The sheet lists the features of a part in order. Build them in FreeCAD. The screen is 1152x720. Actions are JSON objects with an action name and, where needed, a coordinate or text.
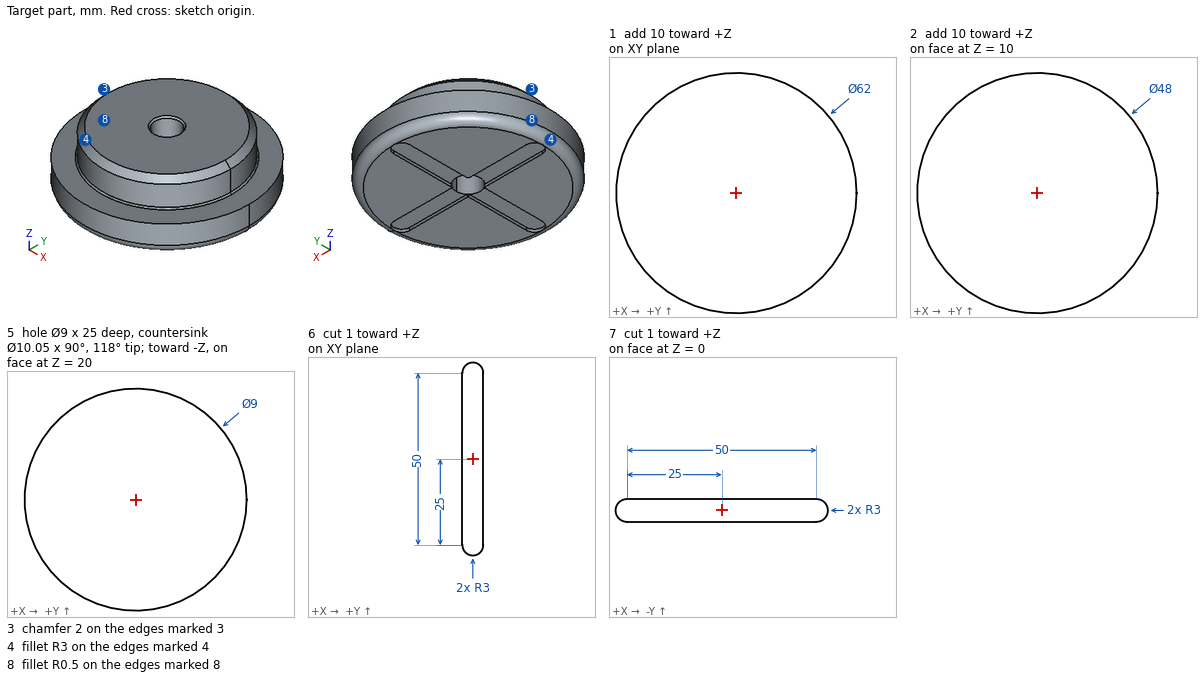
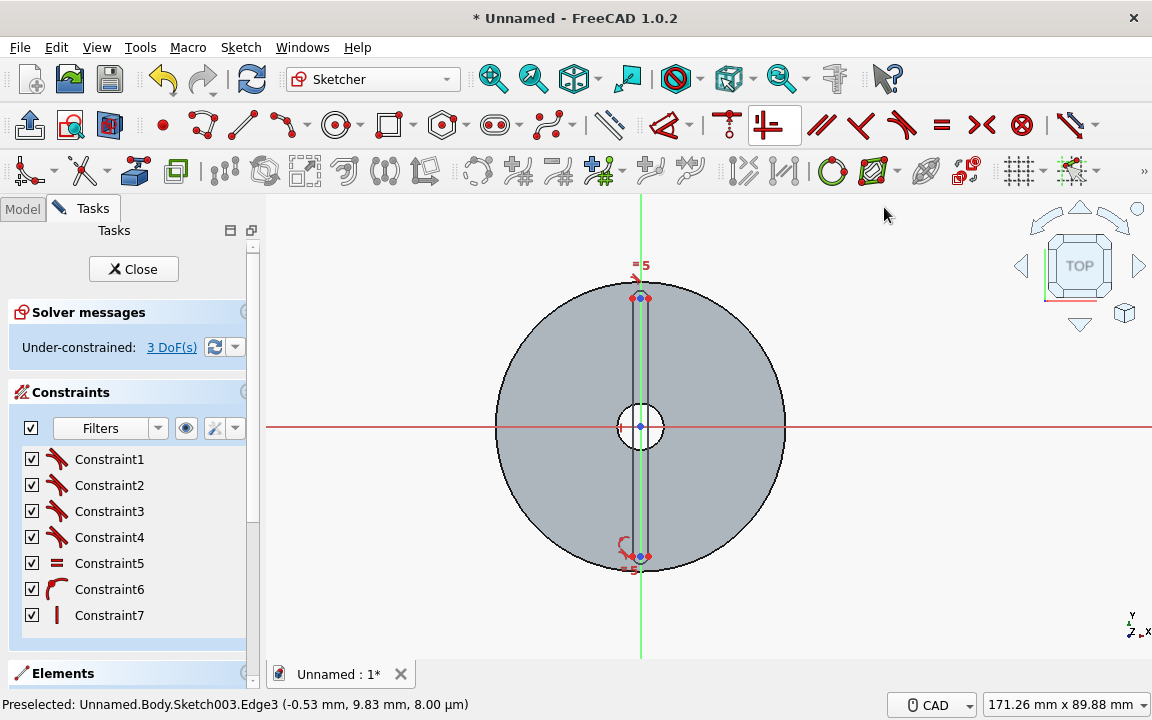
{"action": "key", "text": "d"}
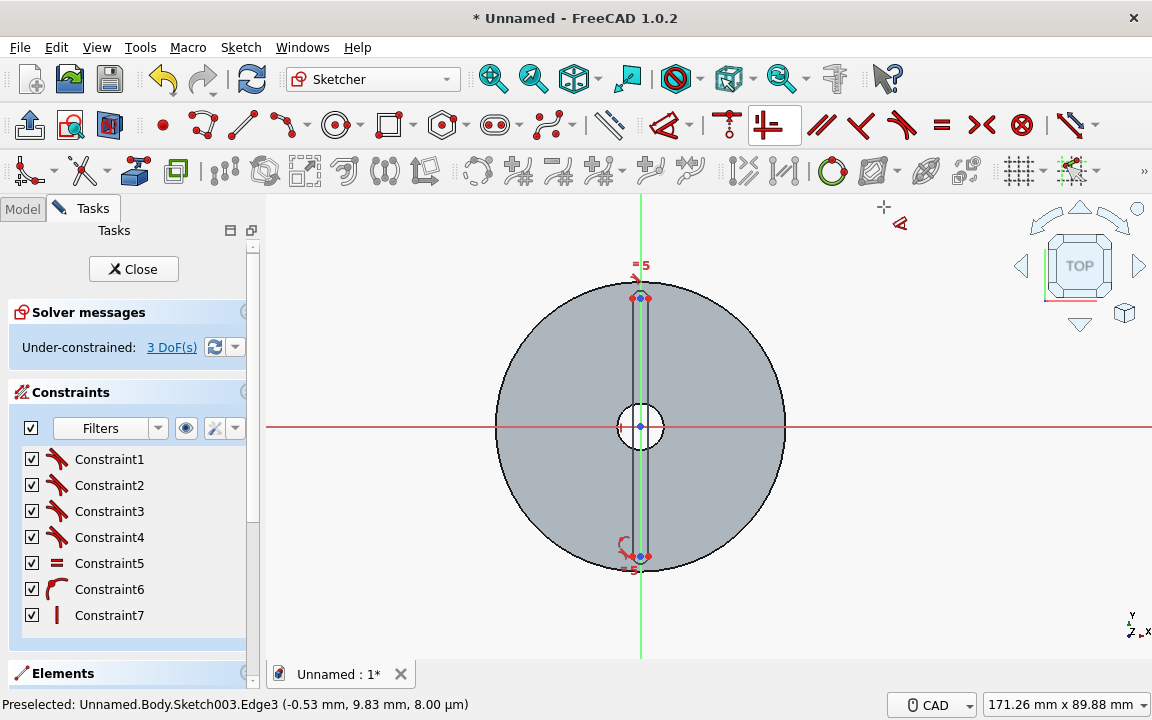
{"action": "scroll", "coordinate": [641, 564], "scroll_direction": "up", "scroll_amount": 5}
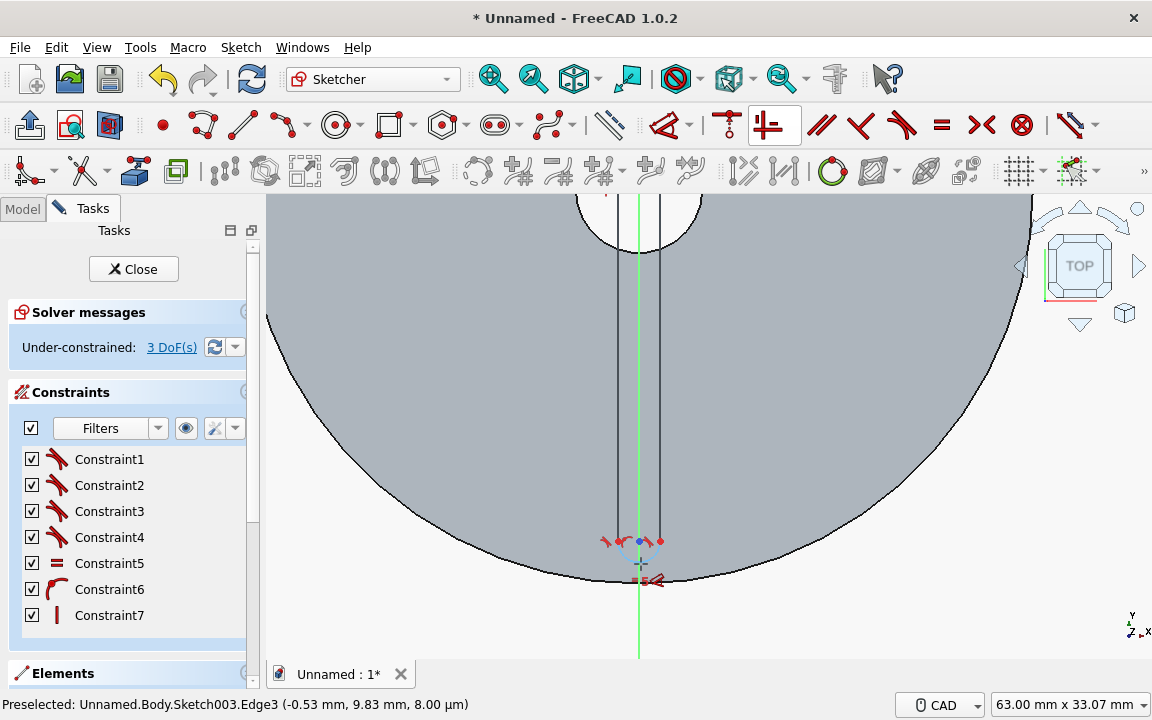
{"action": "left_click", "coordinate": [639, 563]}
{"action": "left_click", "coordinate": [613, 588]}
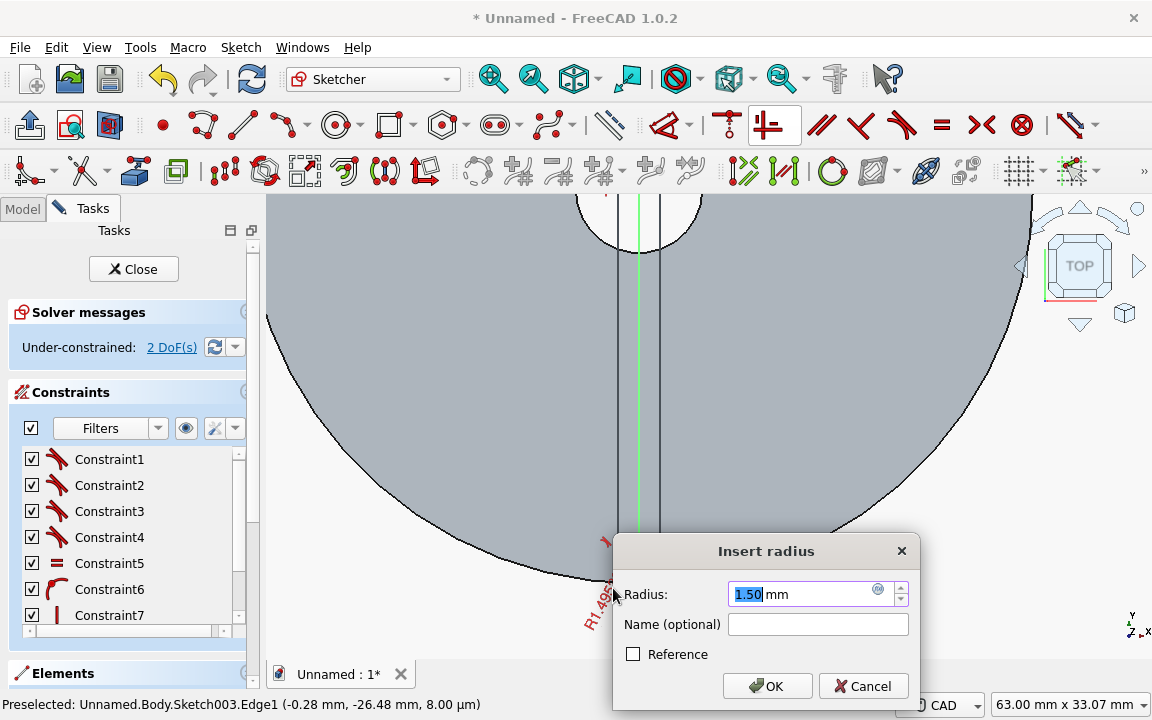
{"action": "type", "text": "3"}
{"action": "key", "text": "Return"}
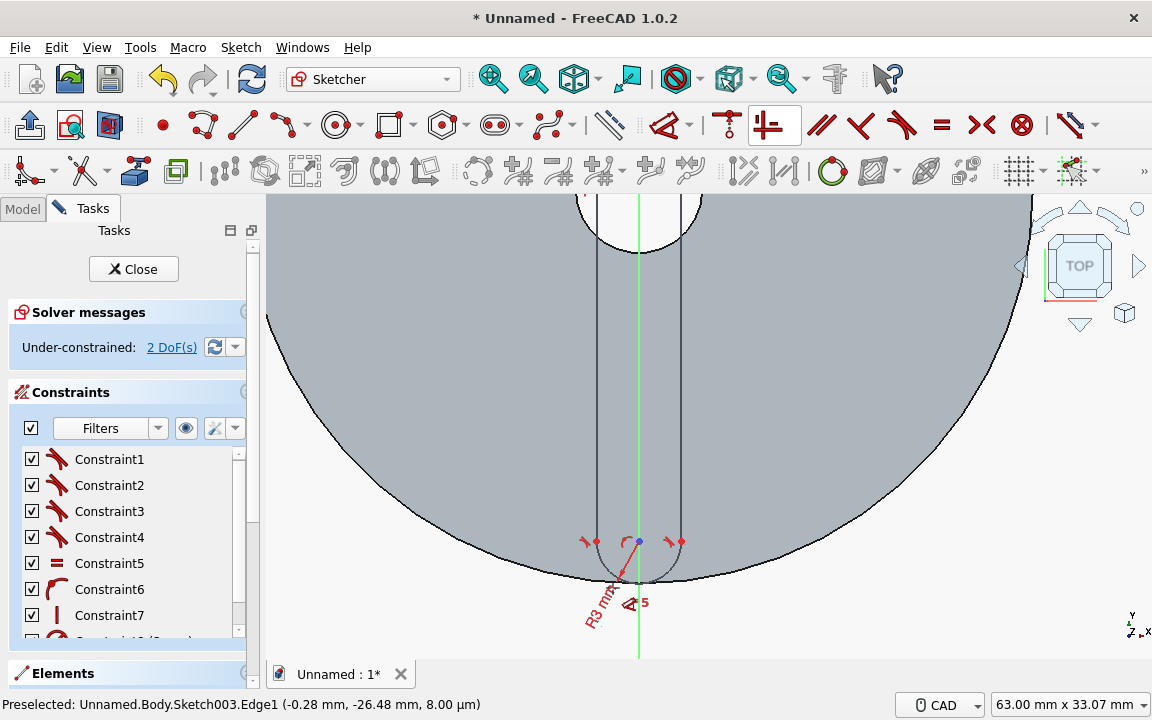
{"action": "left_click", "coordinate": [597, 331]}
{"action": "left_click", "coordinate": [563, 382]}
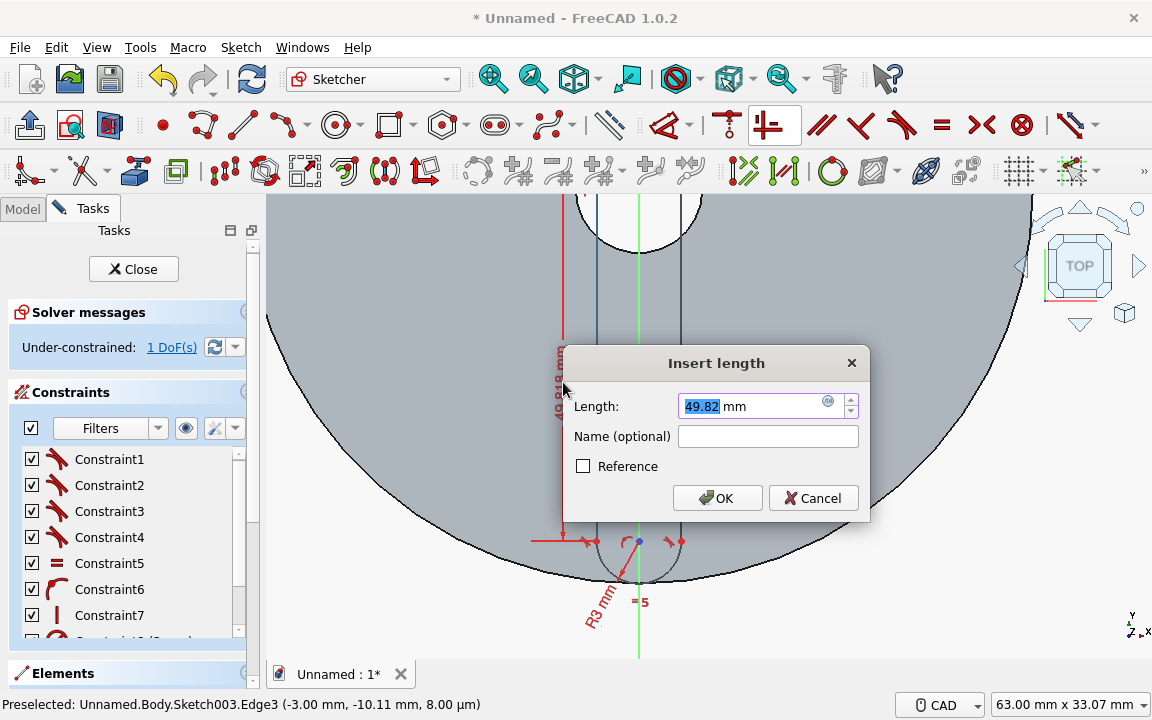
{"action": "type", "text": "50"}
{"action": "key", "text": "Return"}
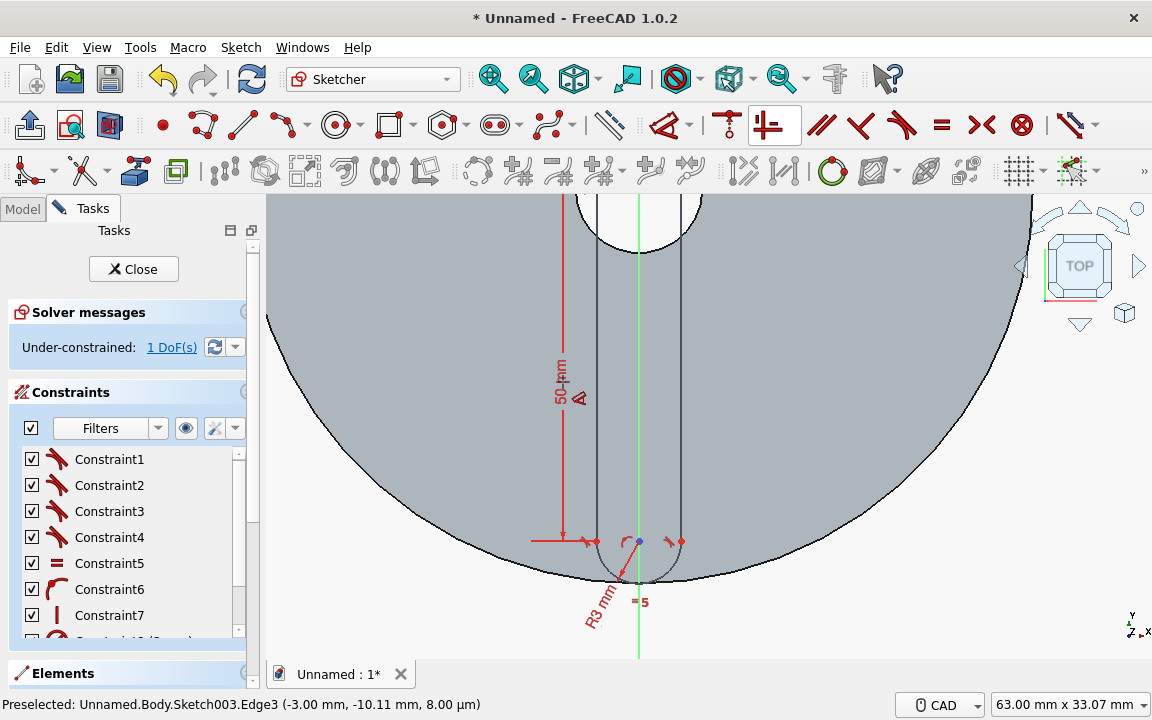
{"action": "left_click", "coordinate": [597, 541]}
{"action": "left_click", "coordinate": [563, 308]}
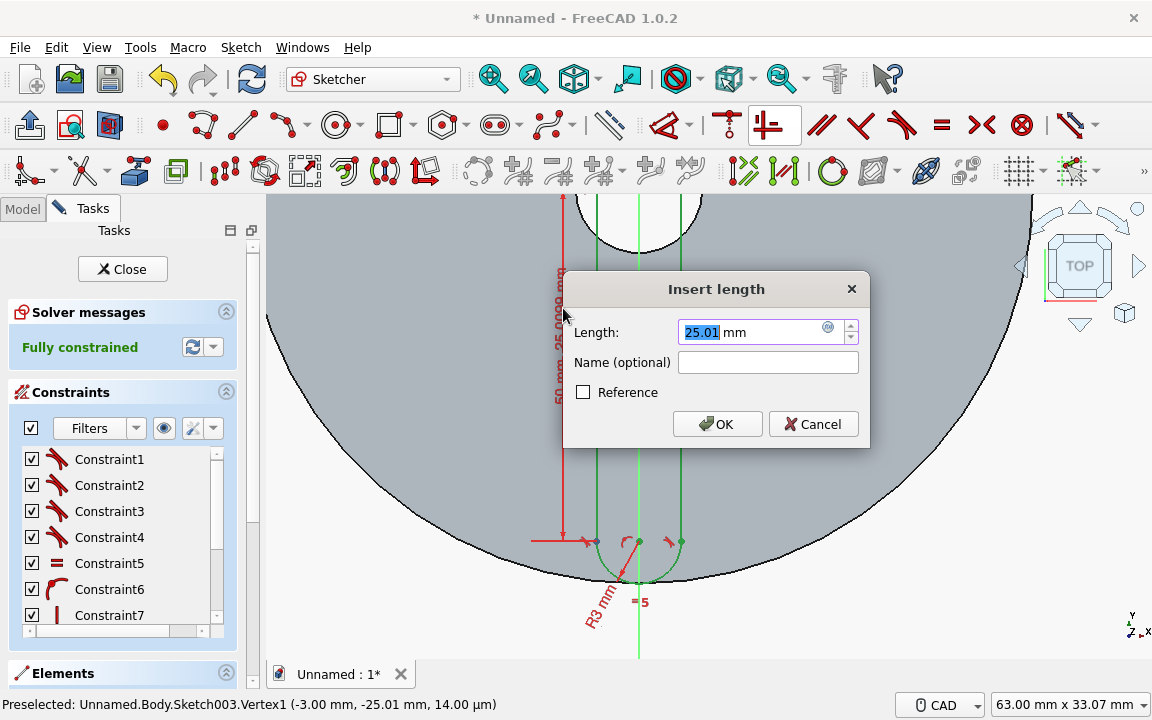
{"action": "type", "text": "25"}
{"action": "key", "text": "Return"}
{"action": "key", "text": "Escape"}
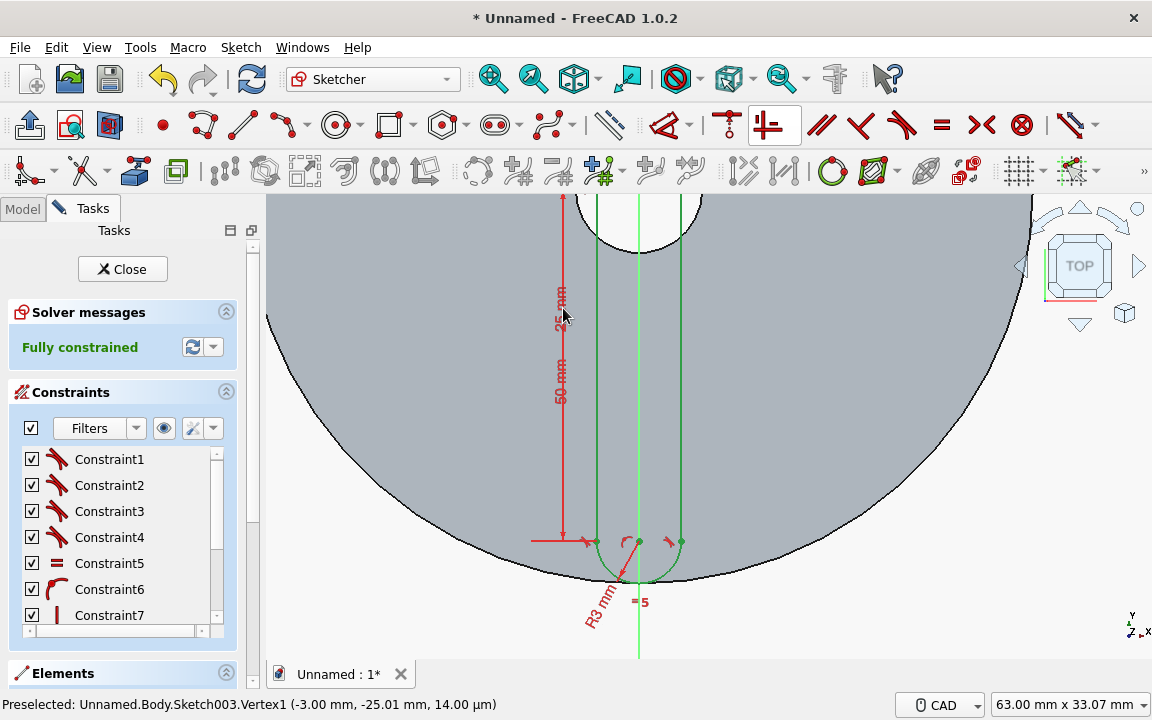
{"action": "left_click", "coordinate": [123, 269]}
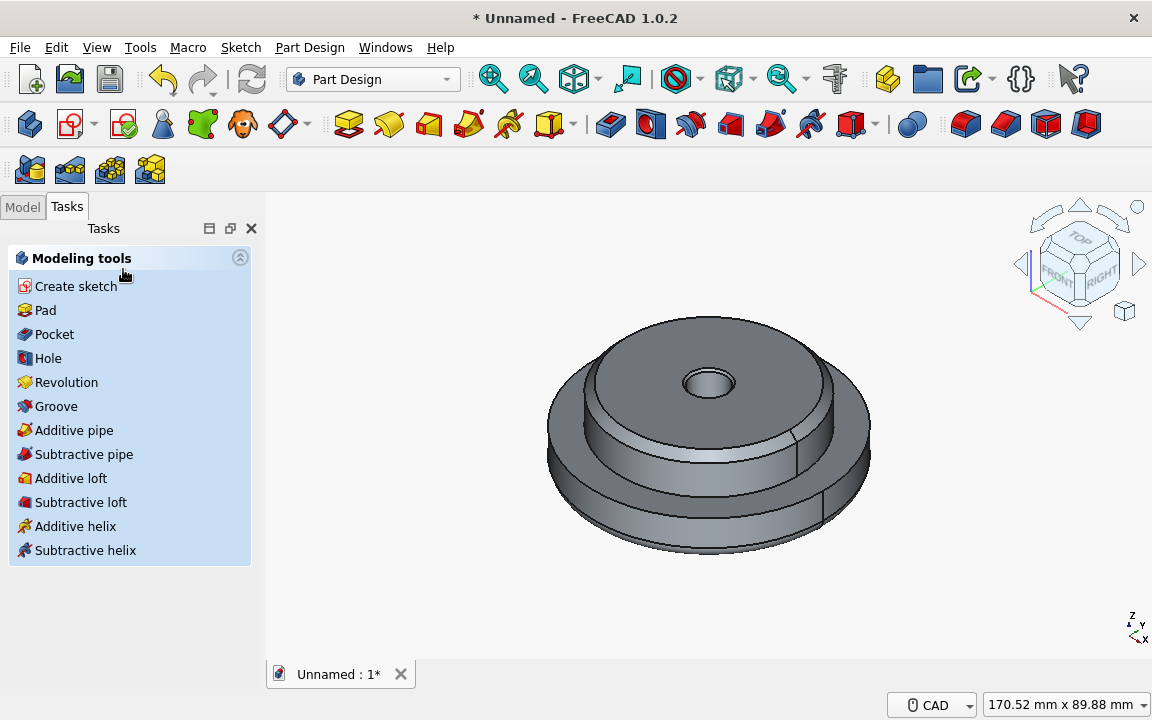
{"action": "left_click", "coordinate": [612, 124]}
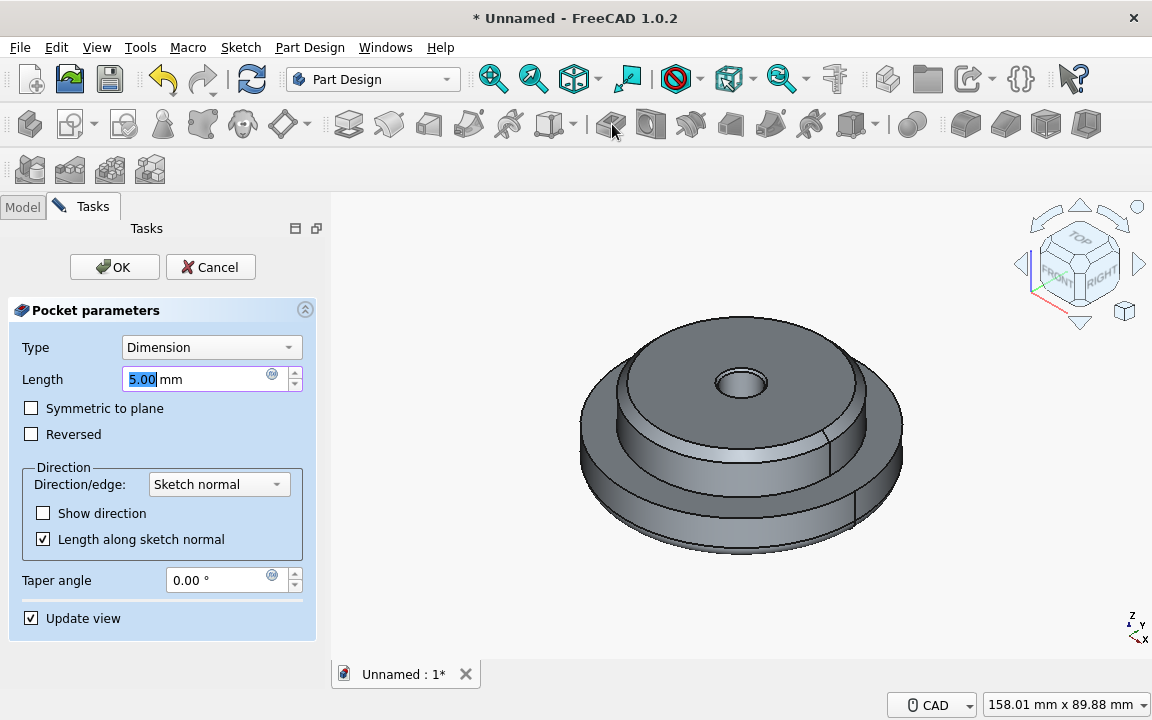
{"action": "type", "text": "1"}
{"action": "key", "text": "Tab"}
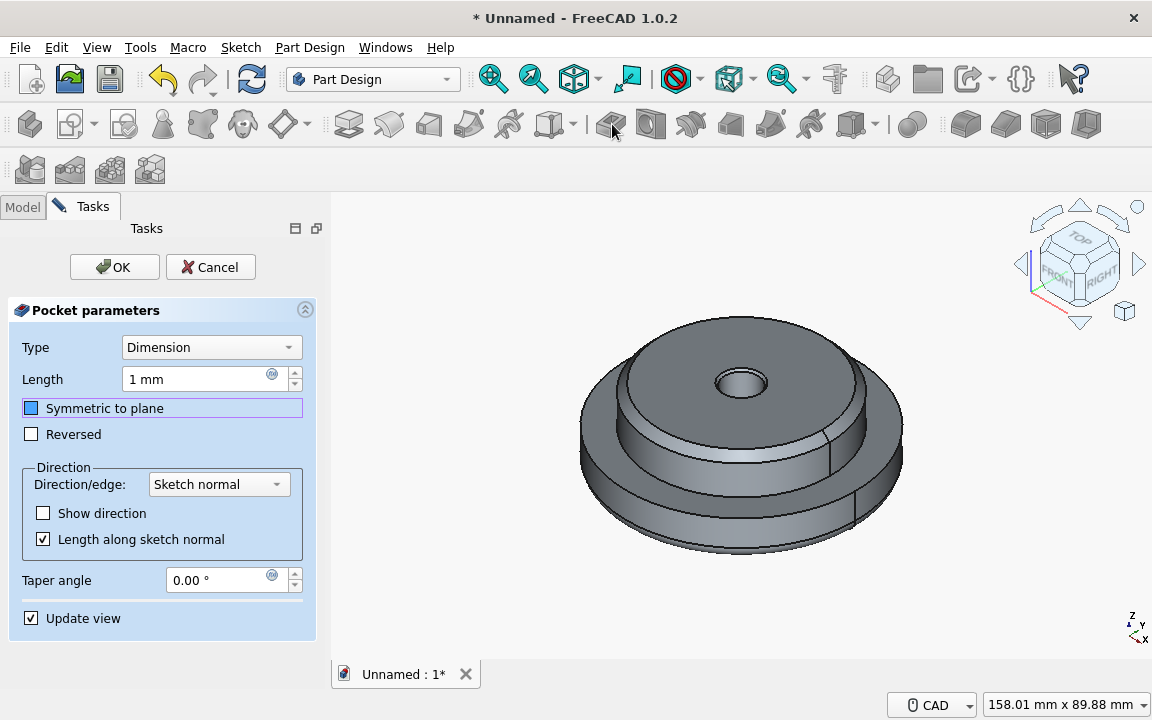
{"action": "left_click", "coordinate": [30, 434]}